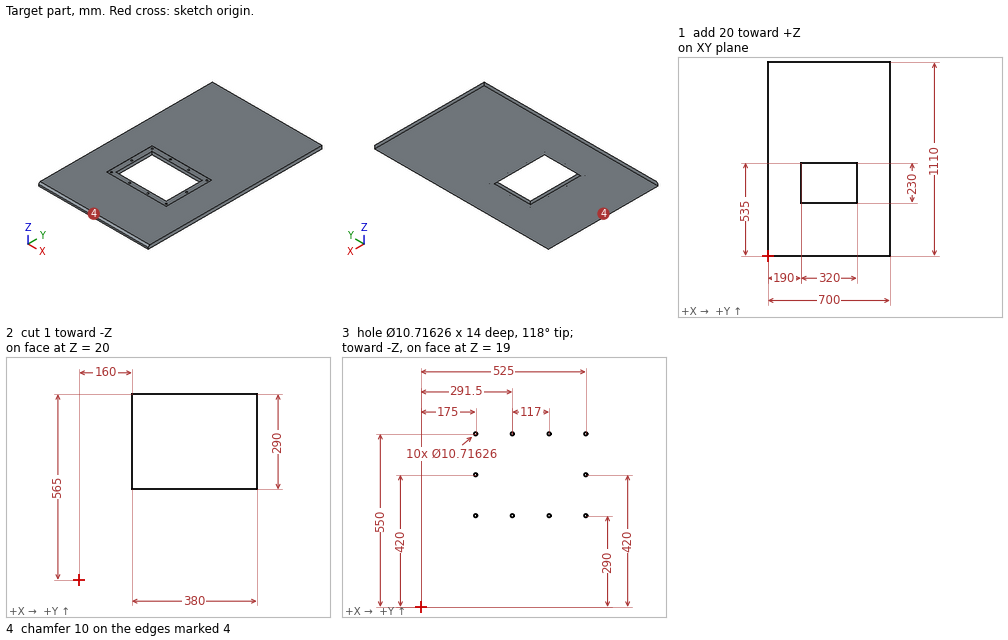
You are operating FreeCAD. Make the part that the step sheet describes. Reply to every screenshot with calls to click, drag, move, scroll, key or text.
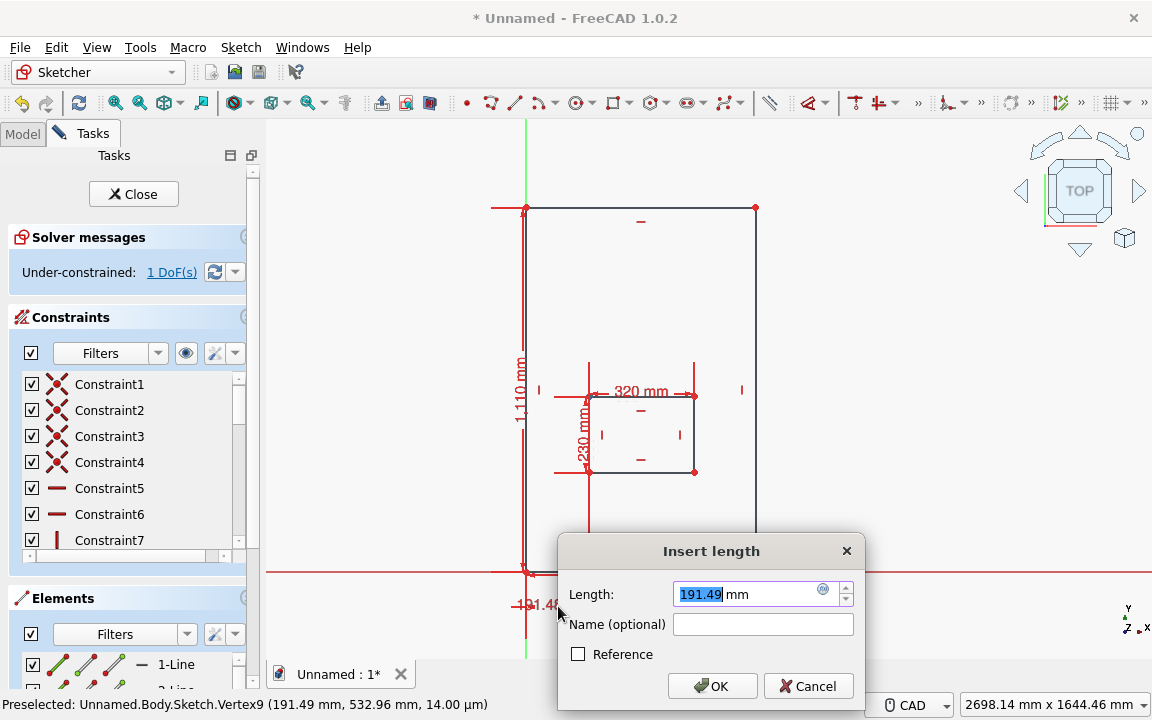
text(190)
key(Return)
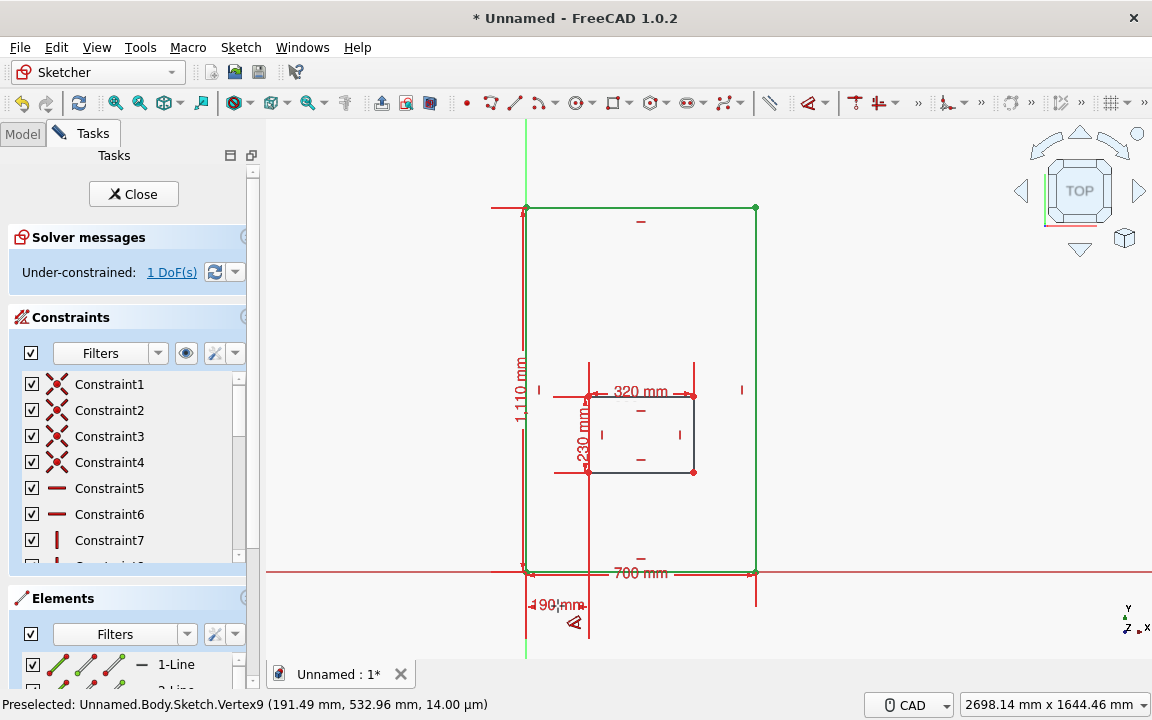
click(589, 397)
click(492, 485)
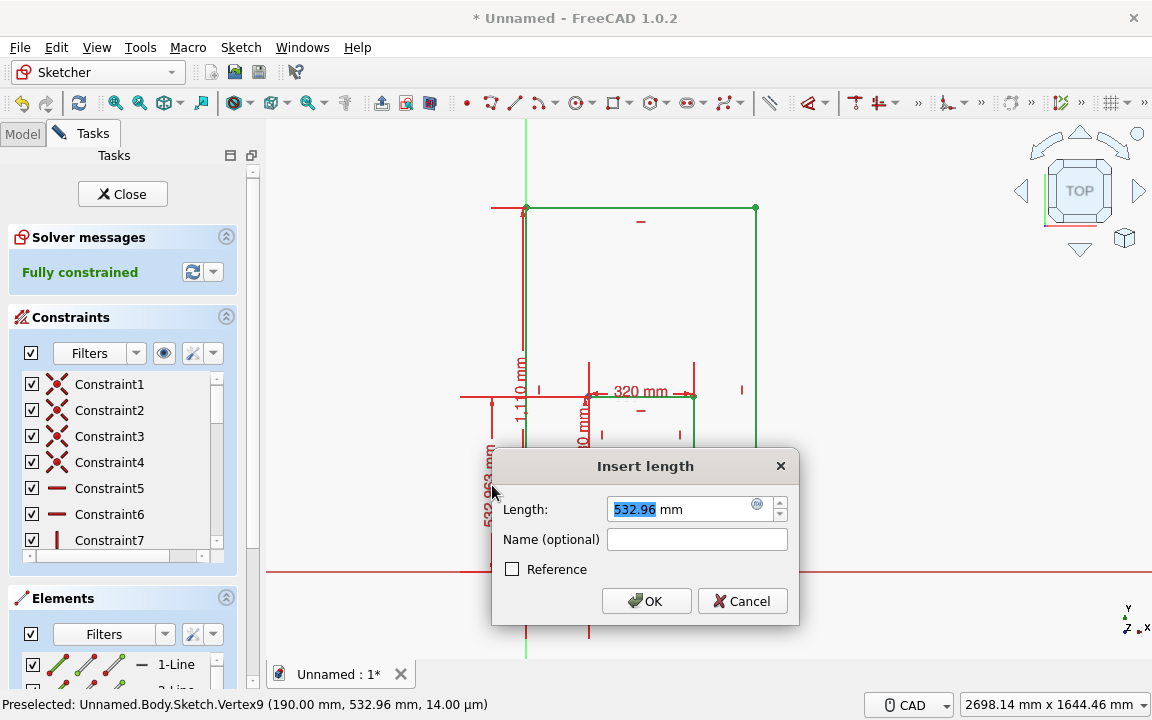
text(535)
key(Return)
key(Escape)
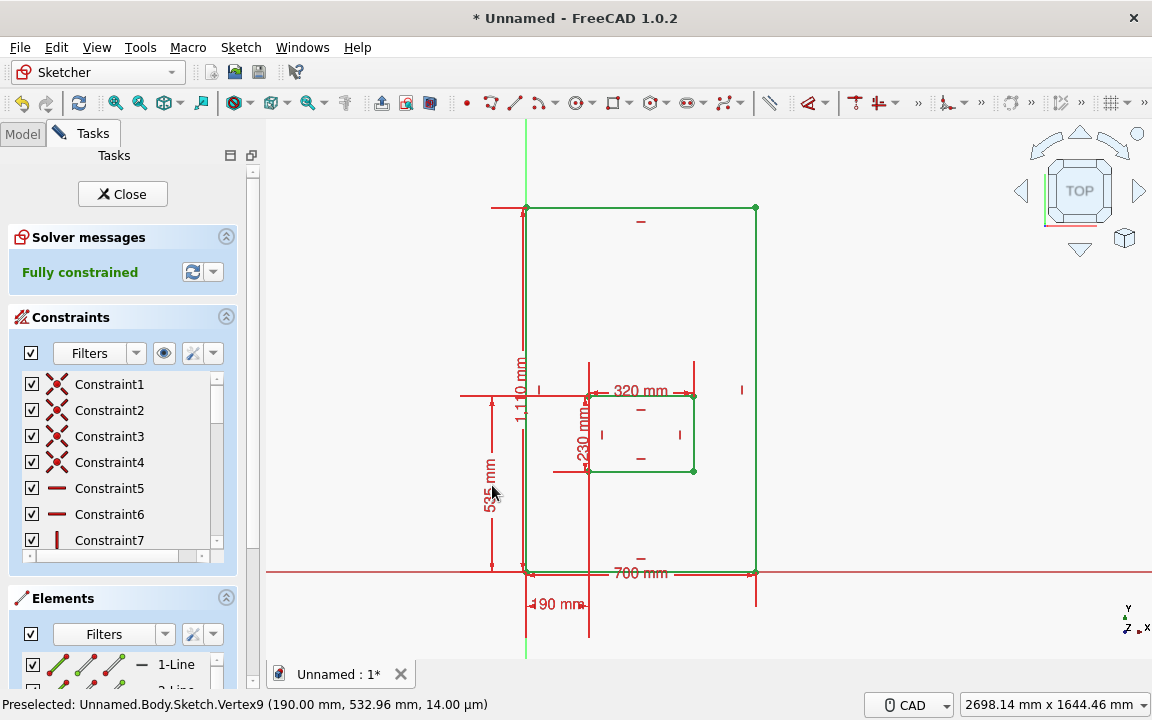
click(123, 194)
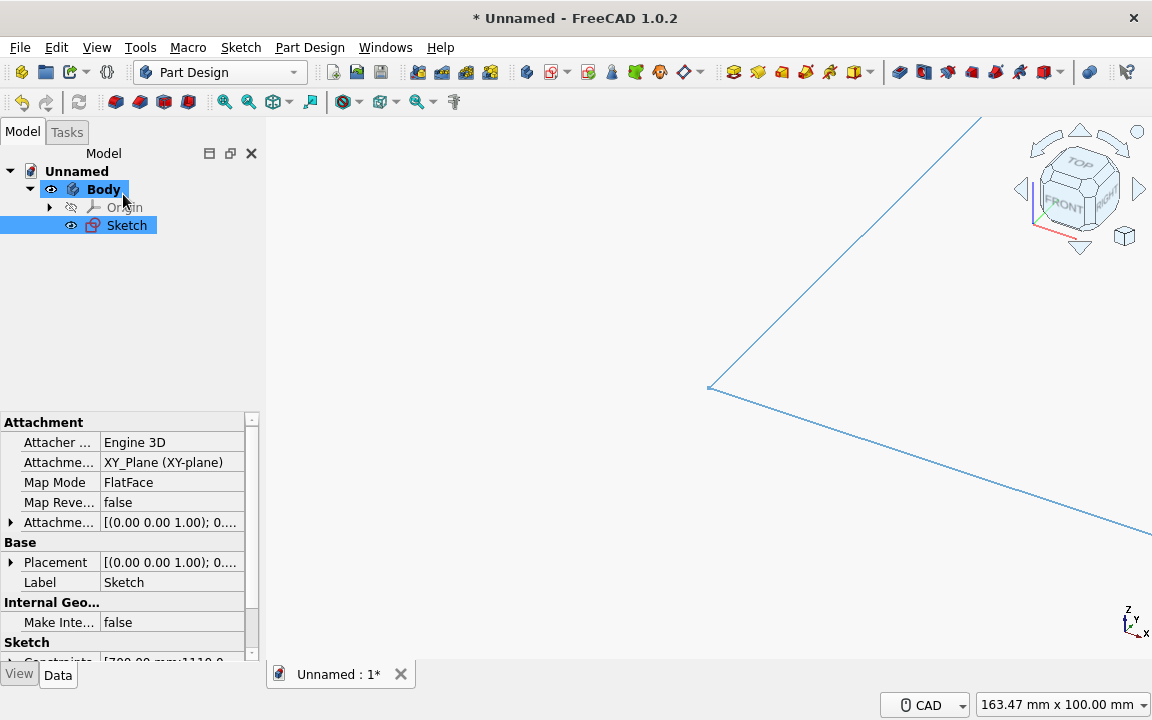
click(734, 72)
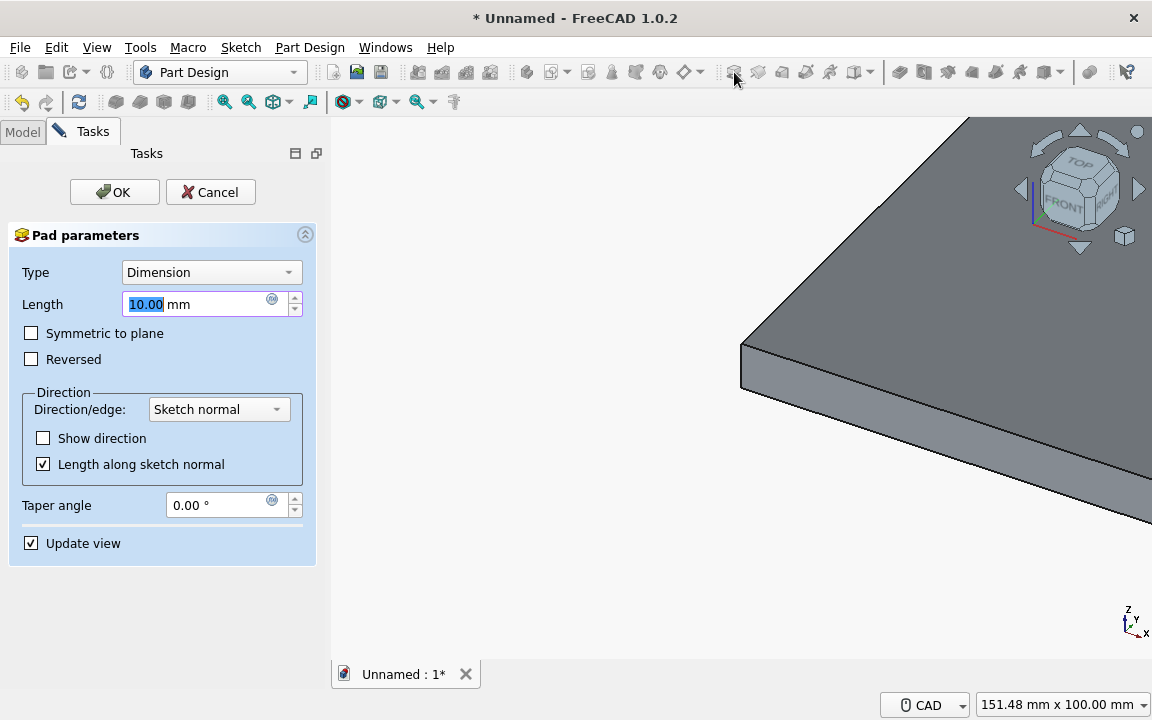
text(20)
key(Tab)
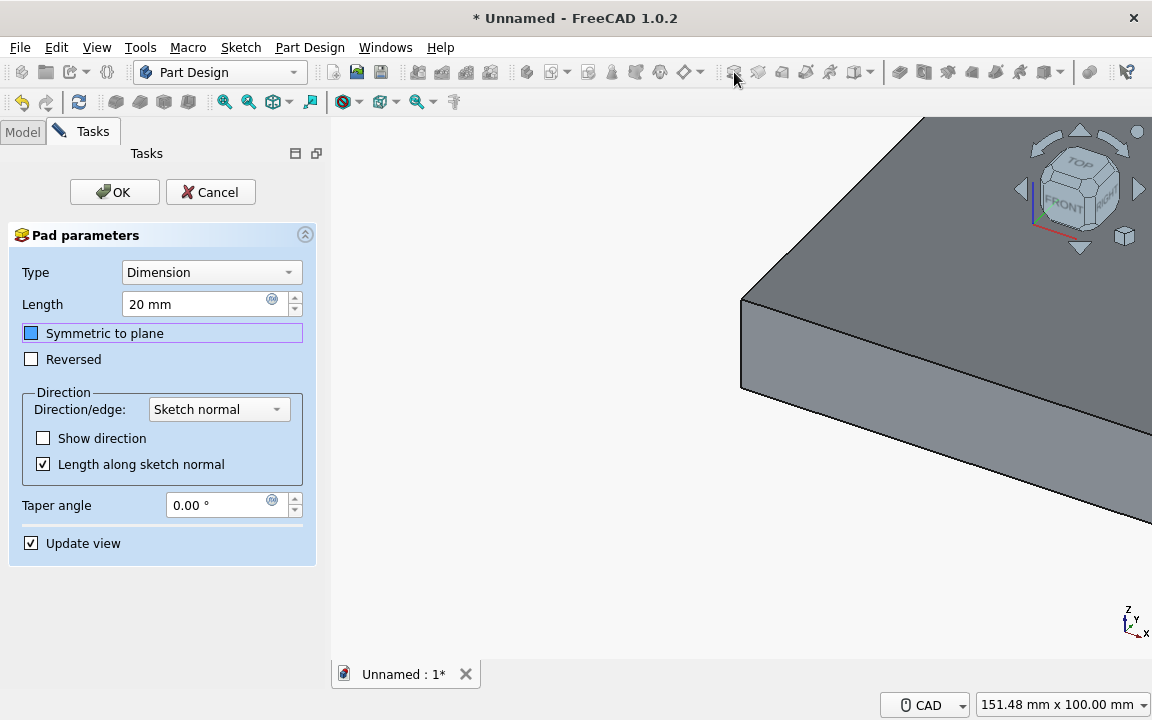
click(115, 192)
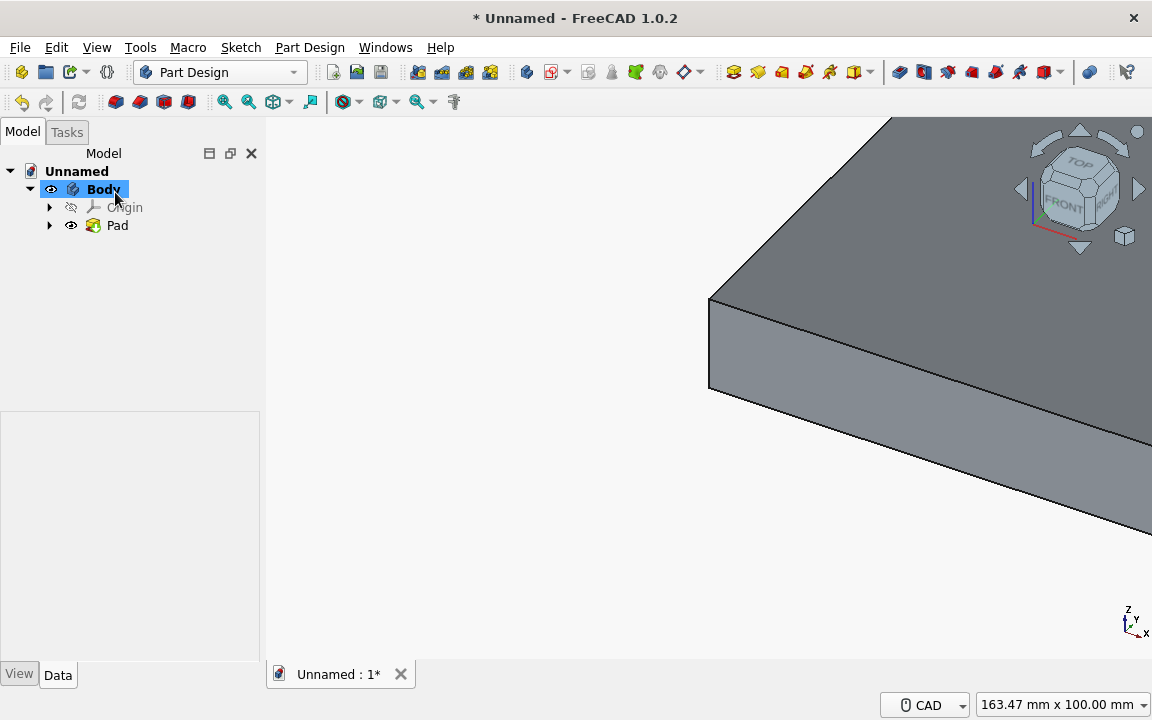
click(226, 102)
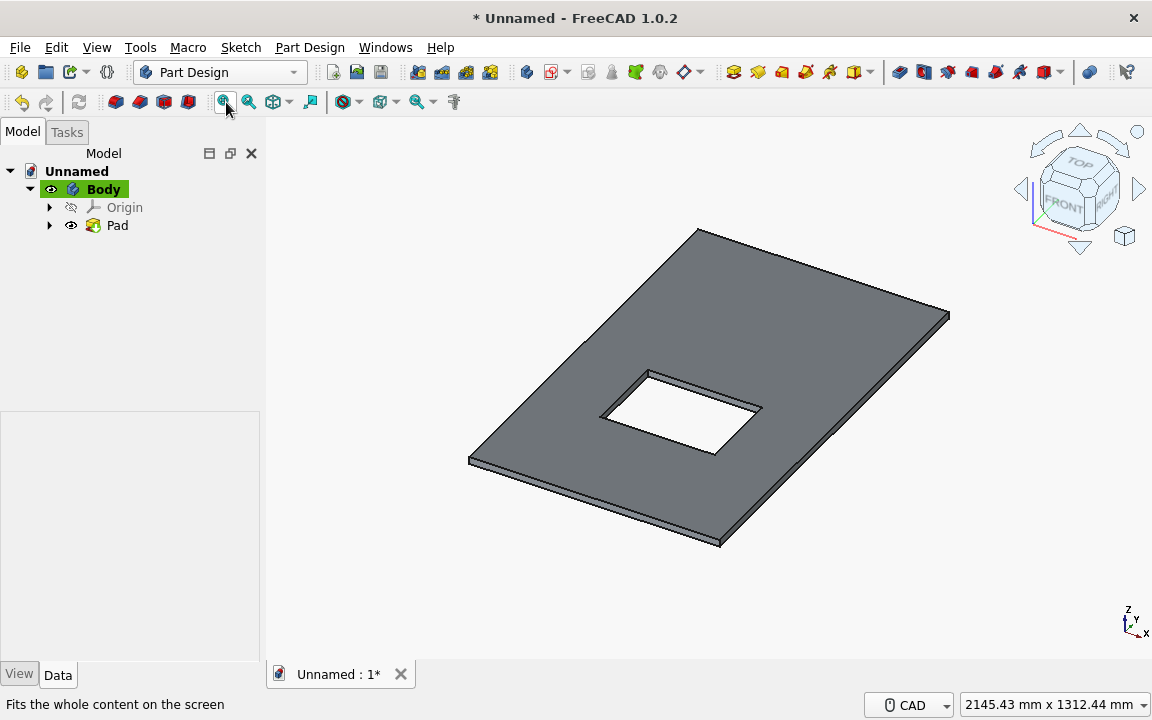
click(810, 330)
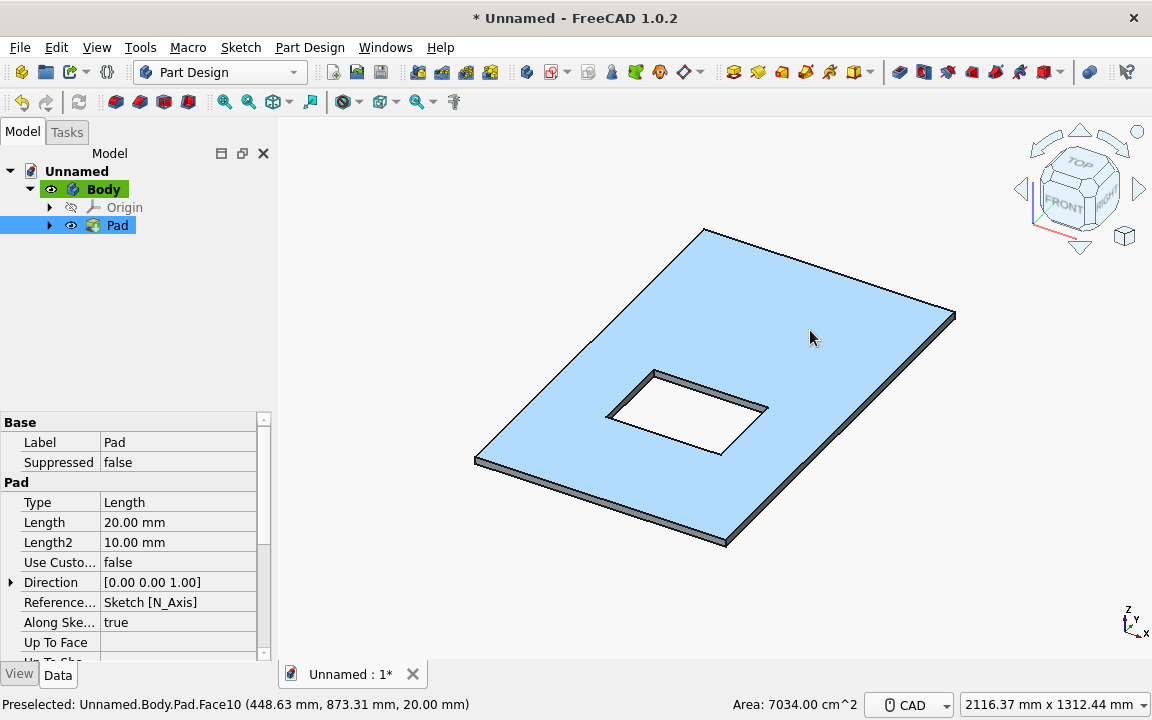
click(552, 72)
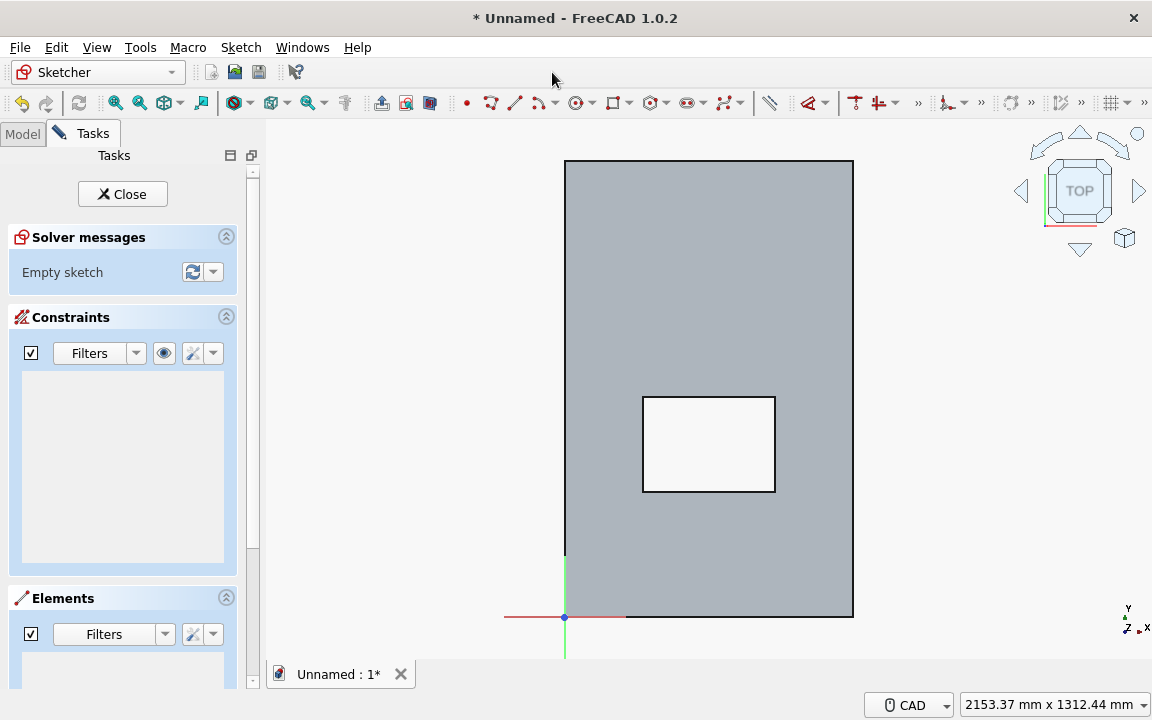
scroll(480, 147, down, 1)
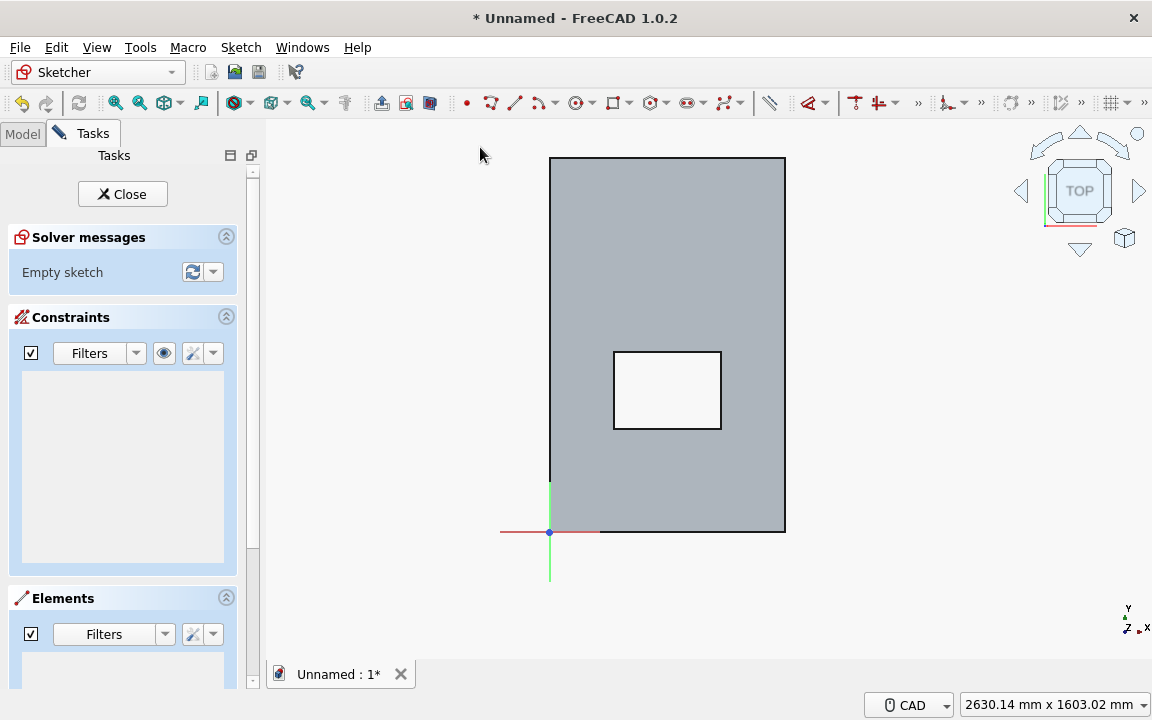
scroll(641, 495, up, 3)